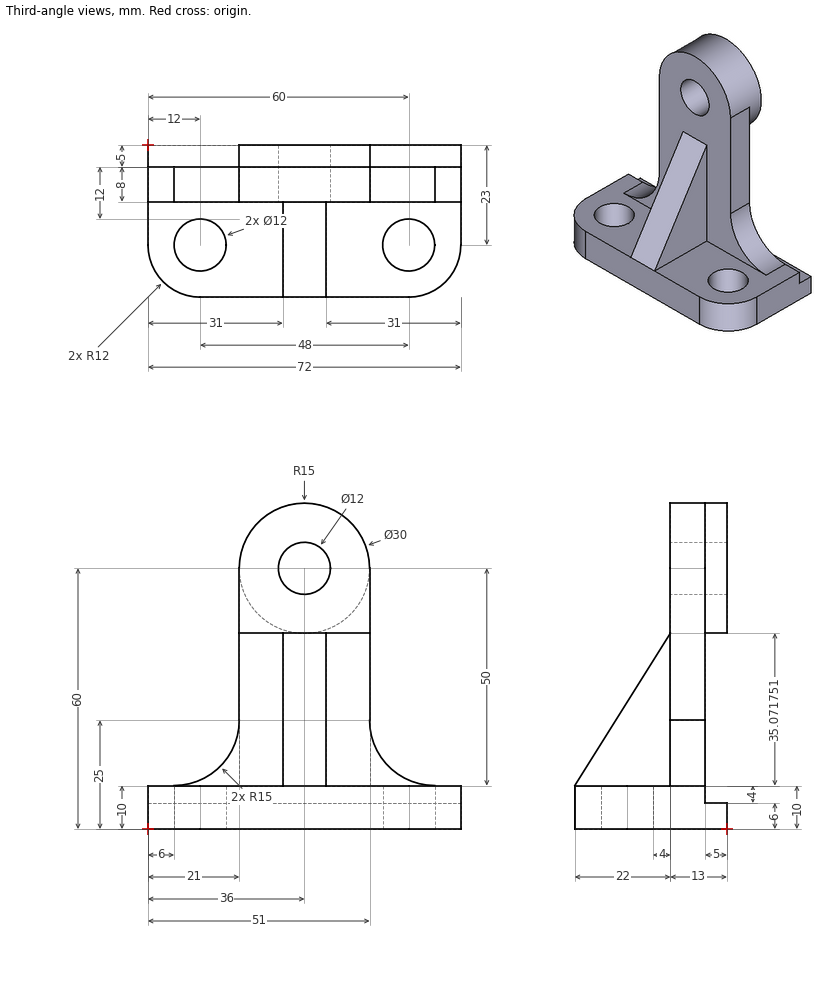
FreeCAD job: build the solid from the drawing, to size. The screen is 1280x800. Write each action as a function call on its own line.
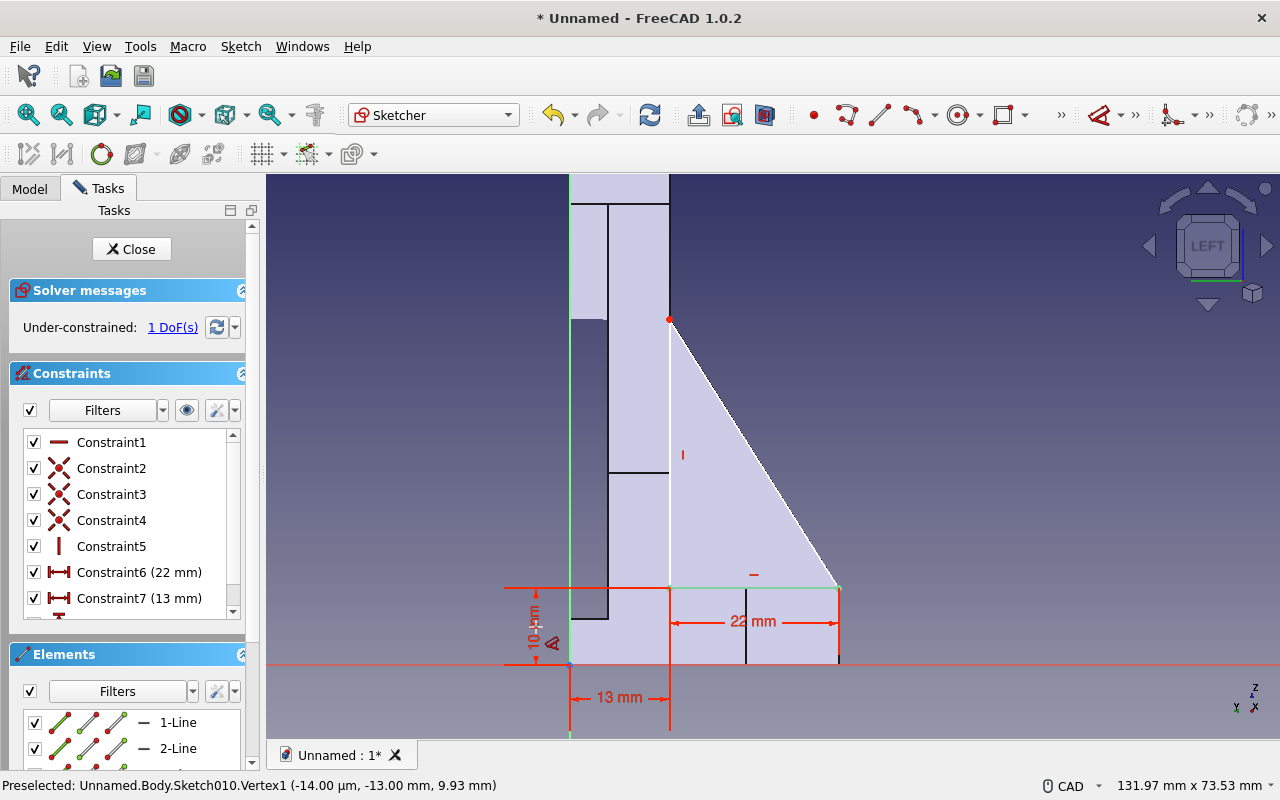
click(670, 401)
click(636, 454)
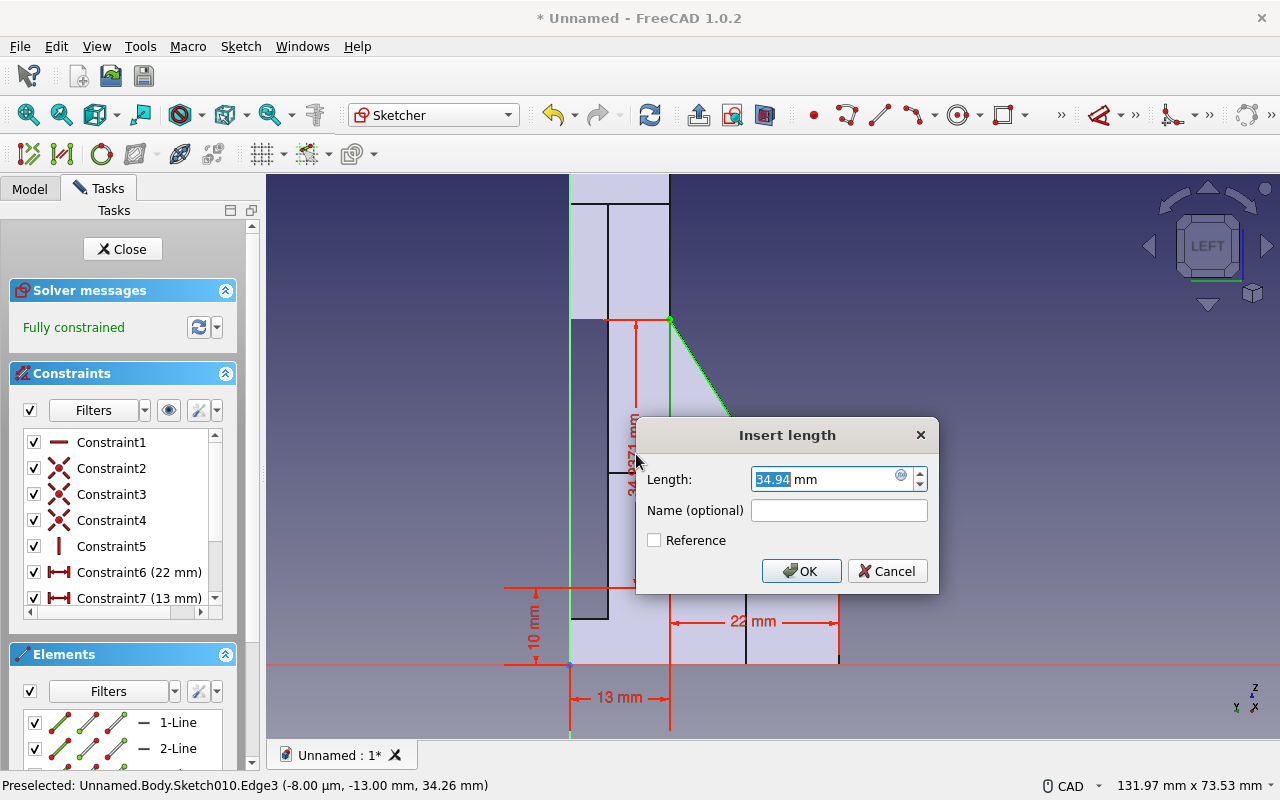
text(35.071751)
key(Return)
key(Escape)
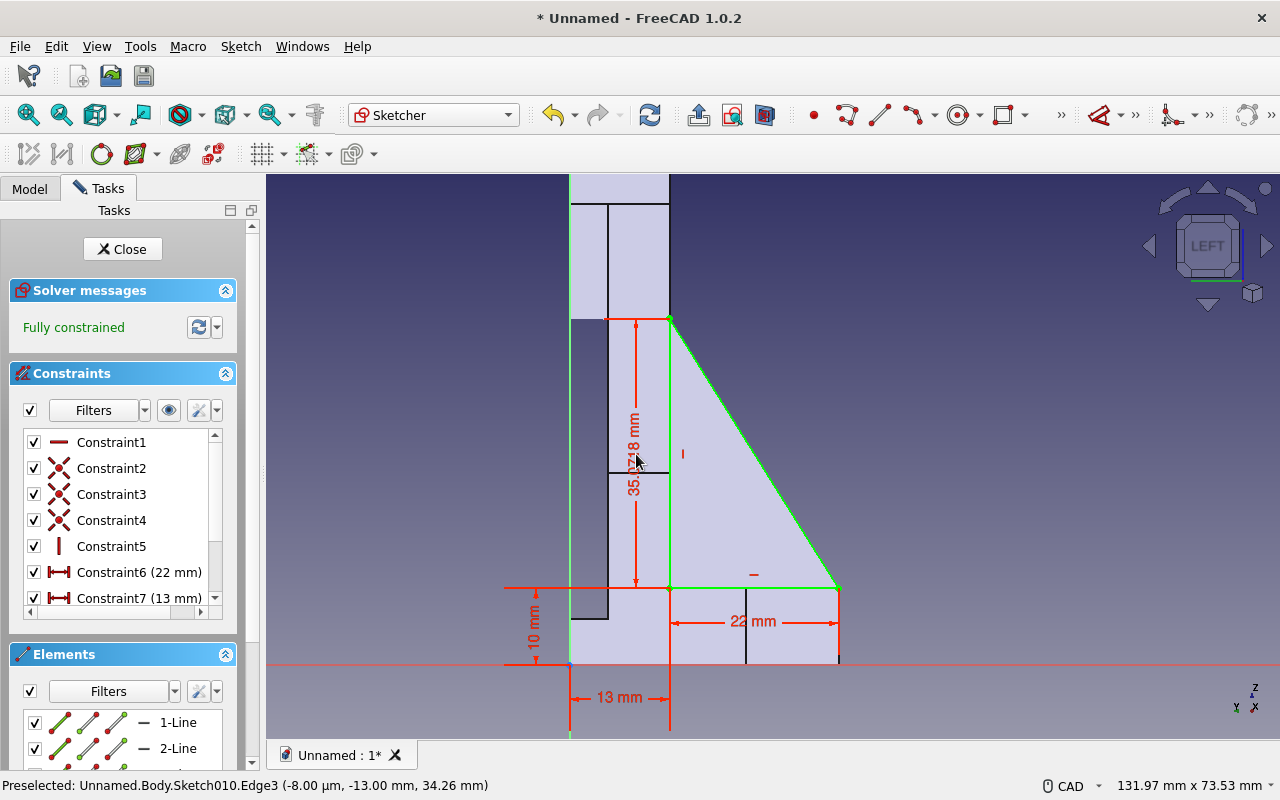
click(123, 249)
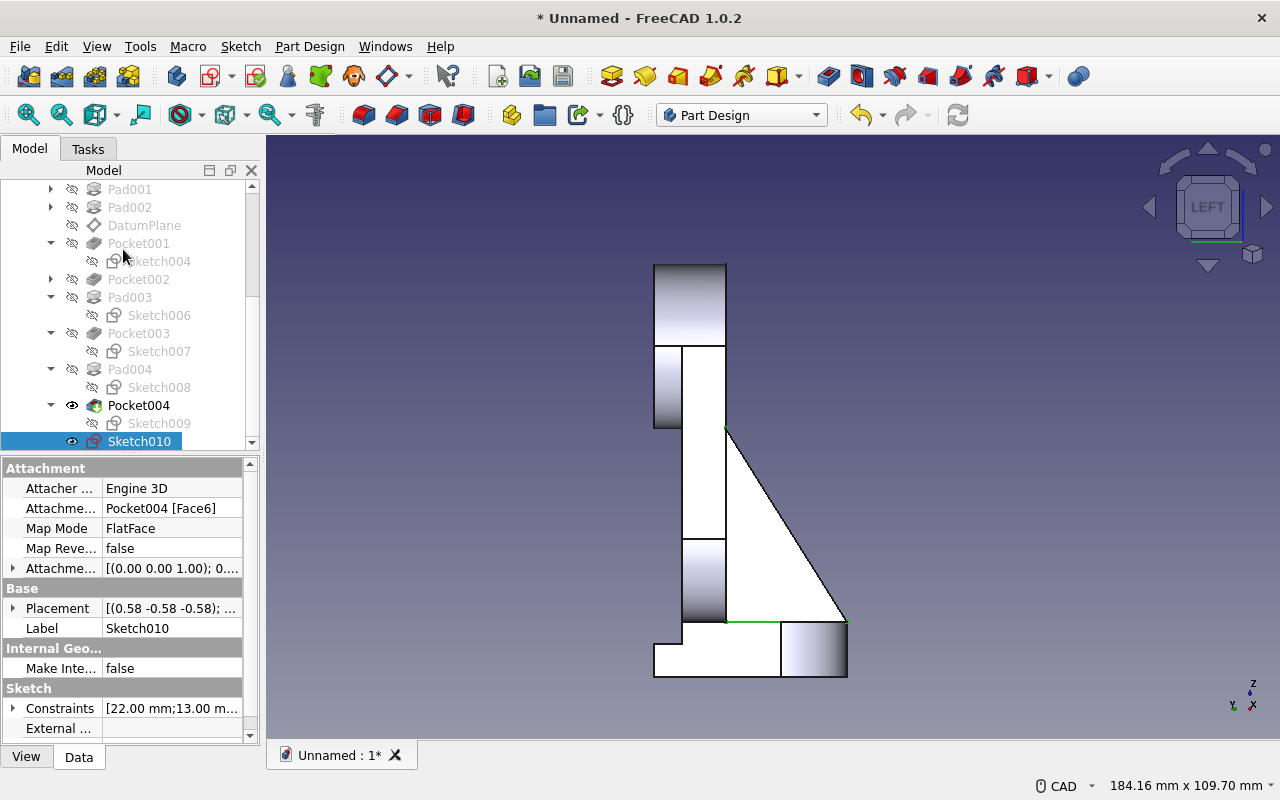
click(829, 76)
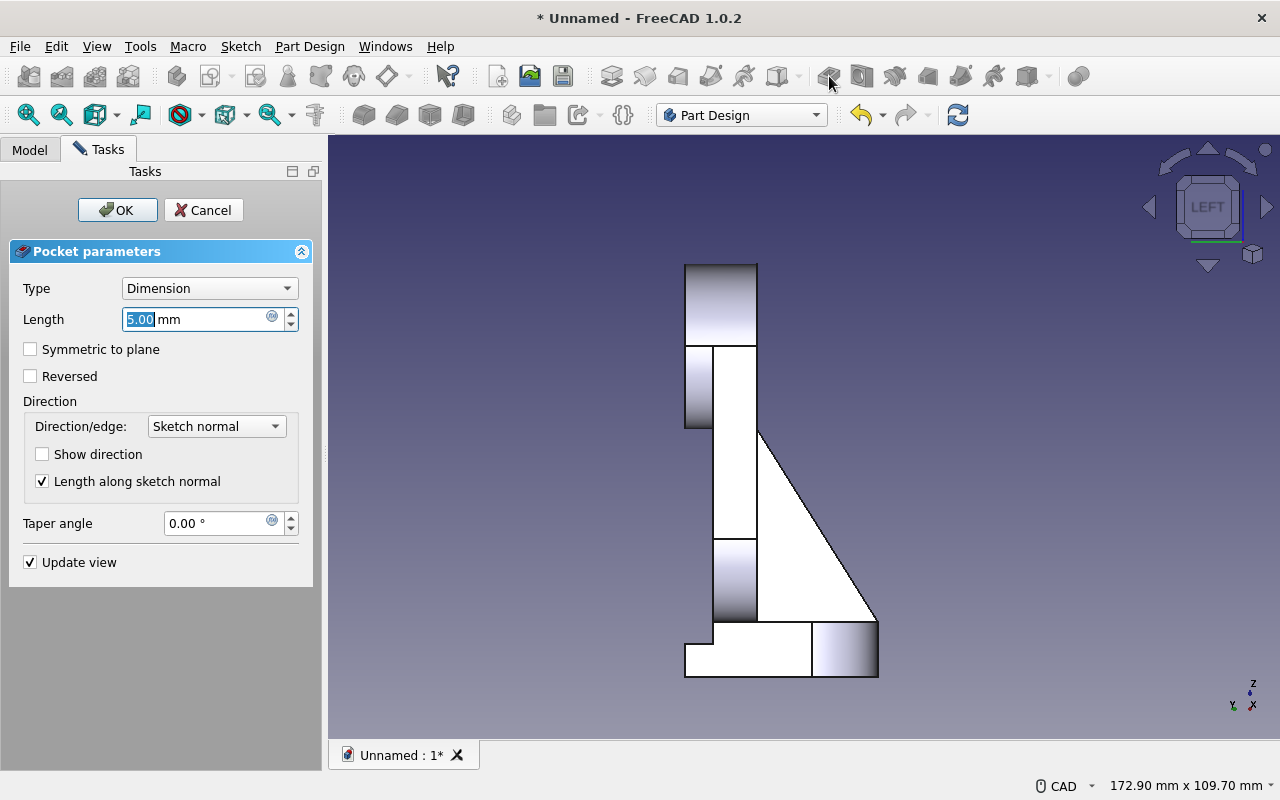
text(31)
key(Tab)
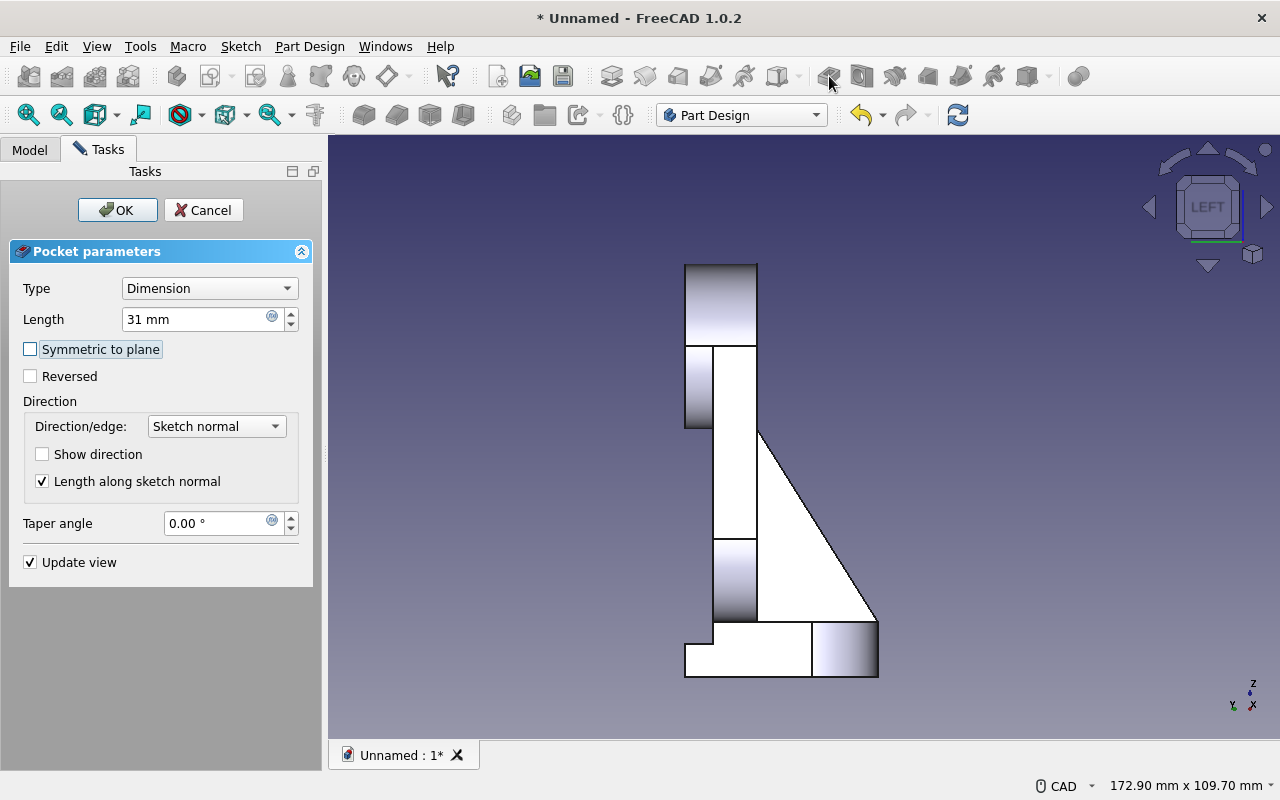
click(118, 210)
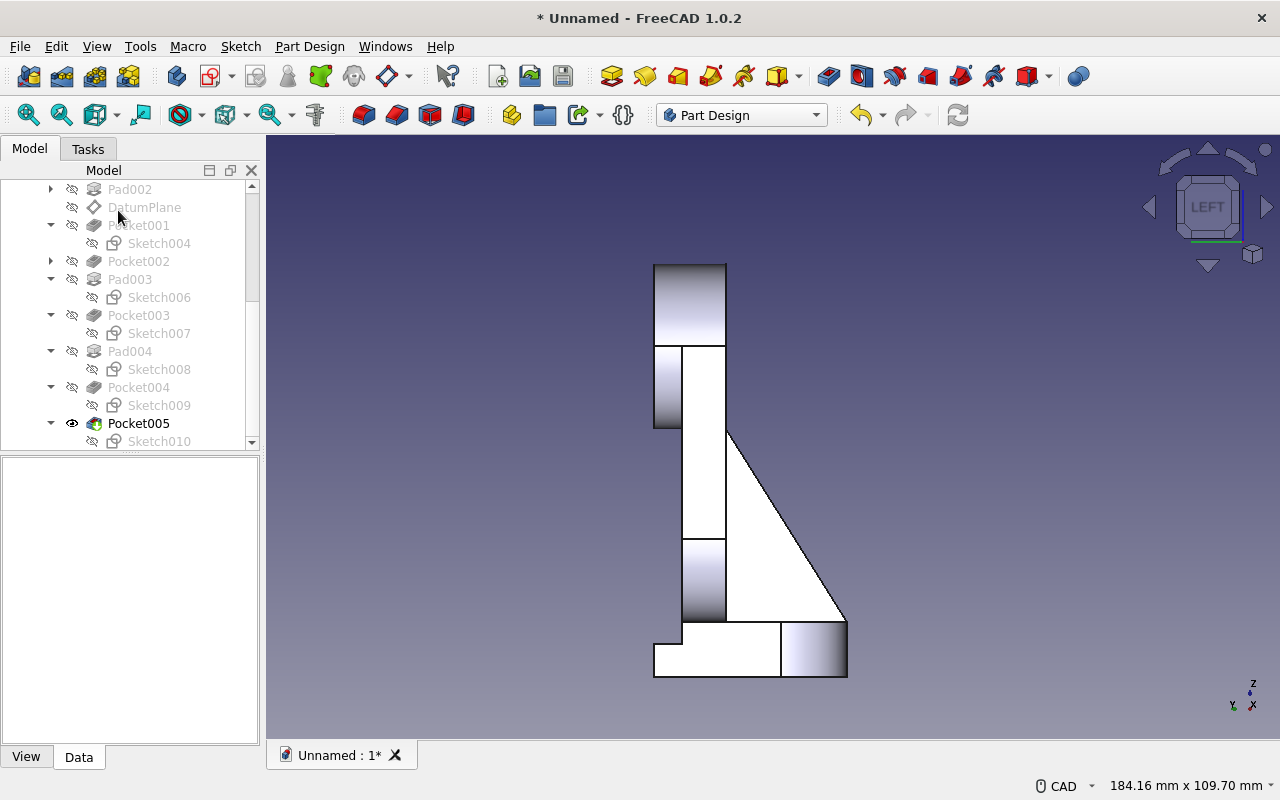
key(0)